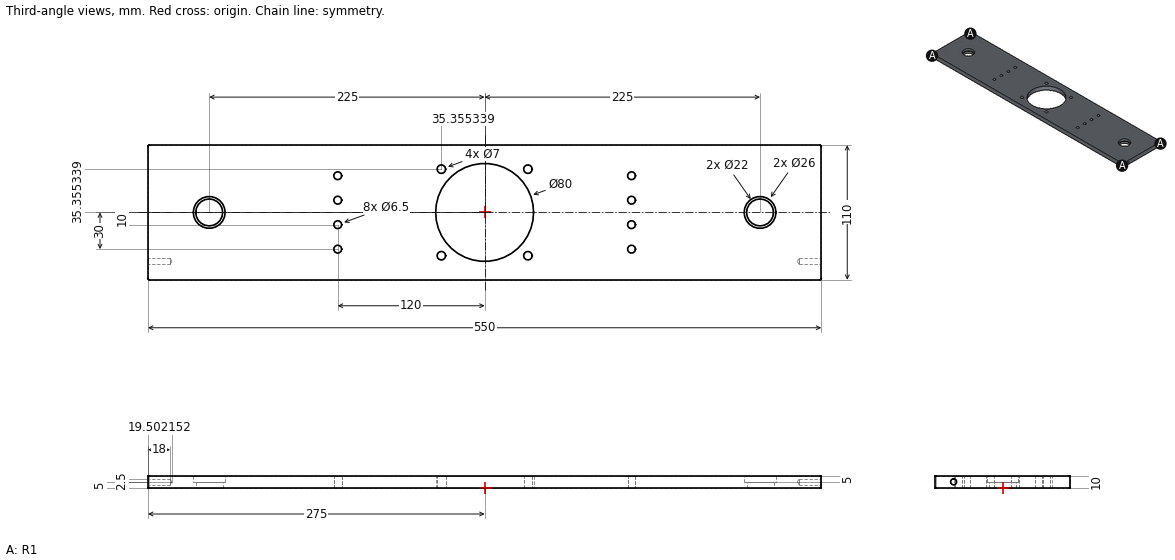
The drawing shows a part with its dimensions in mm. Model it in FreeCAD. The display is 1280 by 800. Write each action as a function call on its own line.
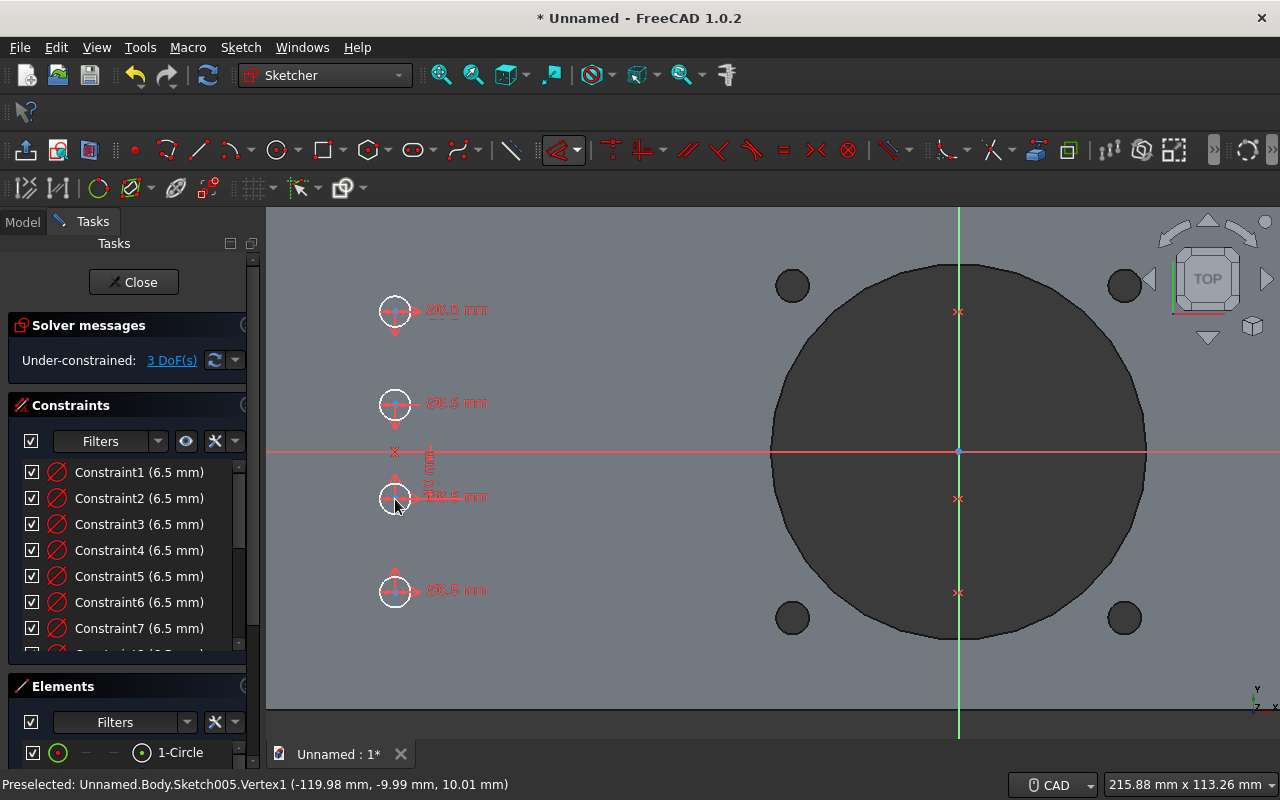
click(395, 592)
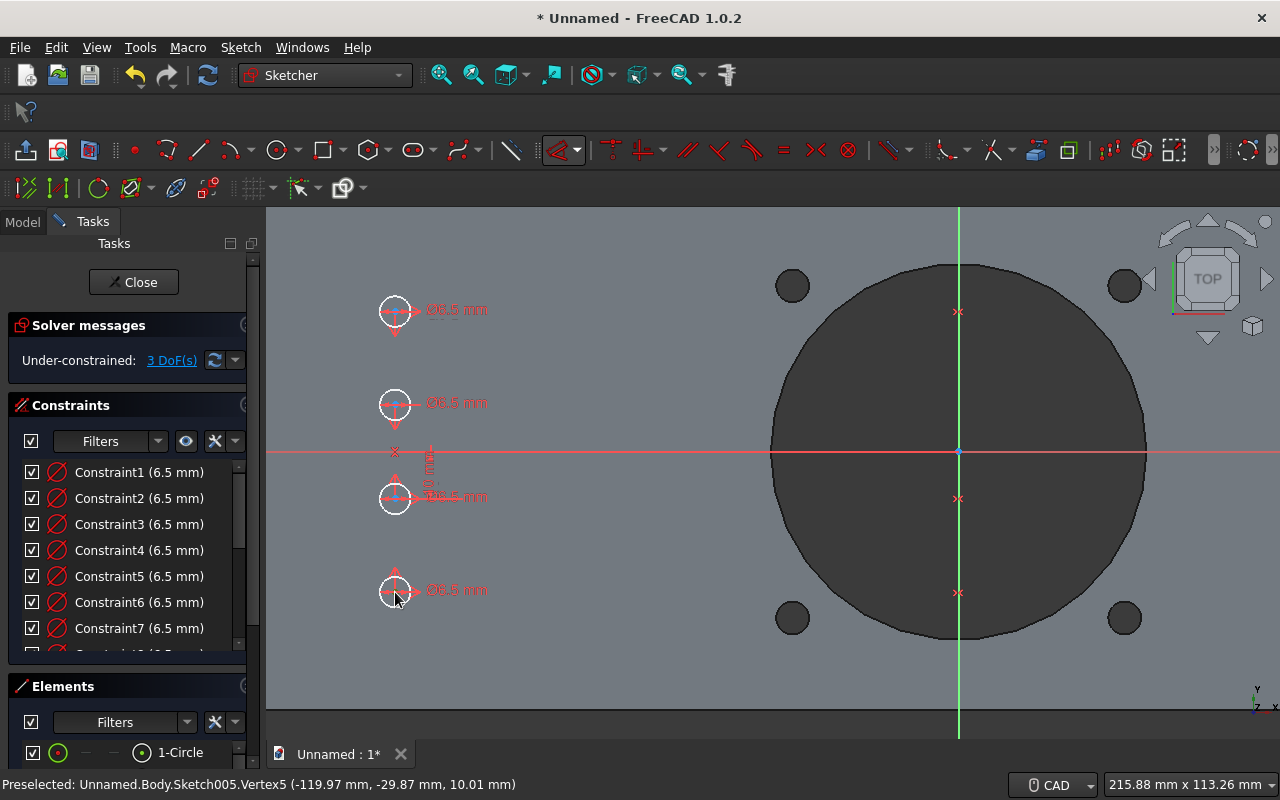
key(i)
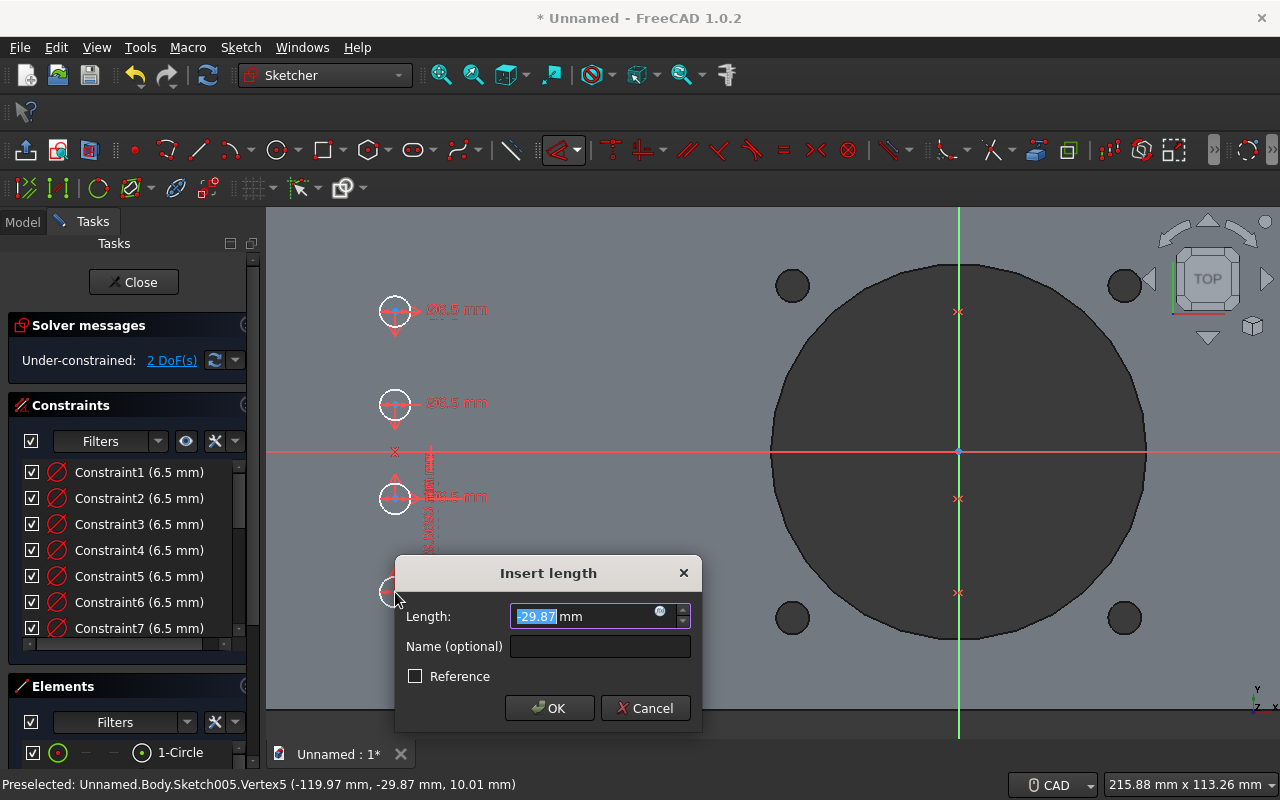
text(-30)
key(Return)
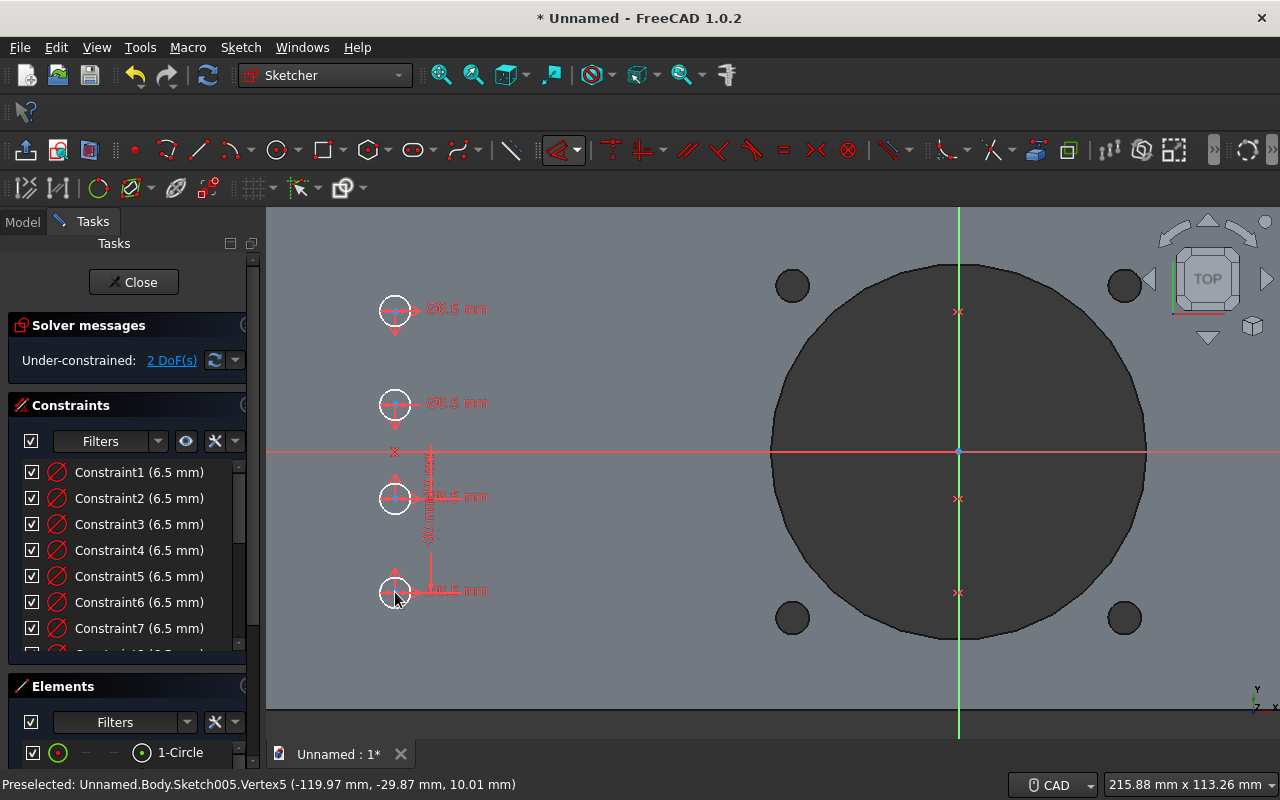
click(395, 499)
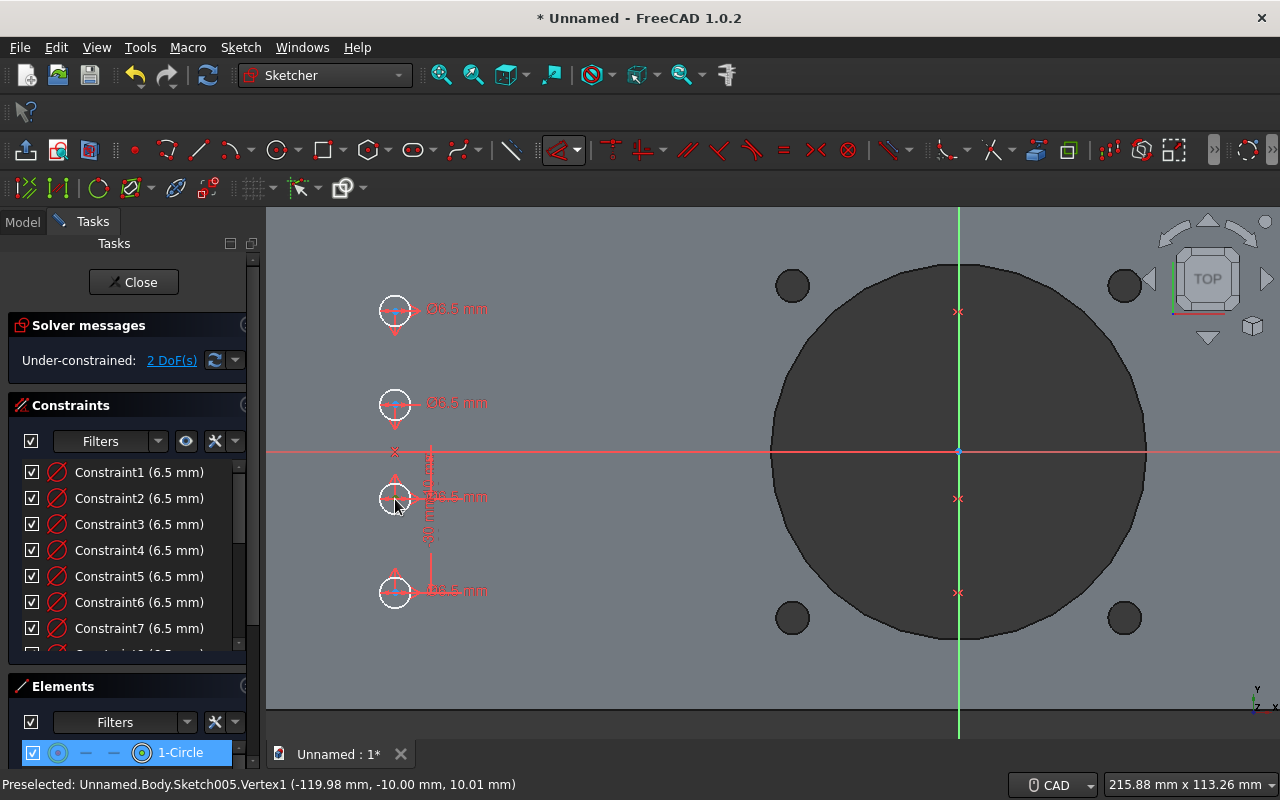
click(580, 150)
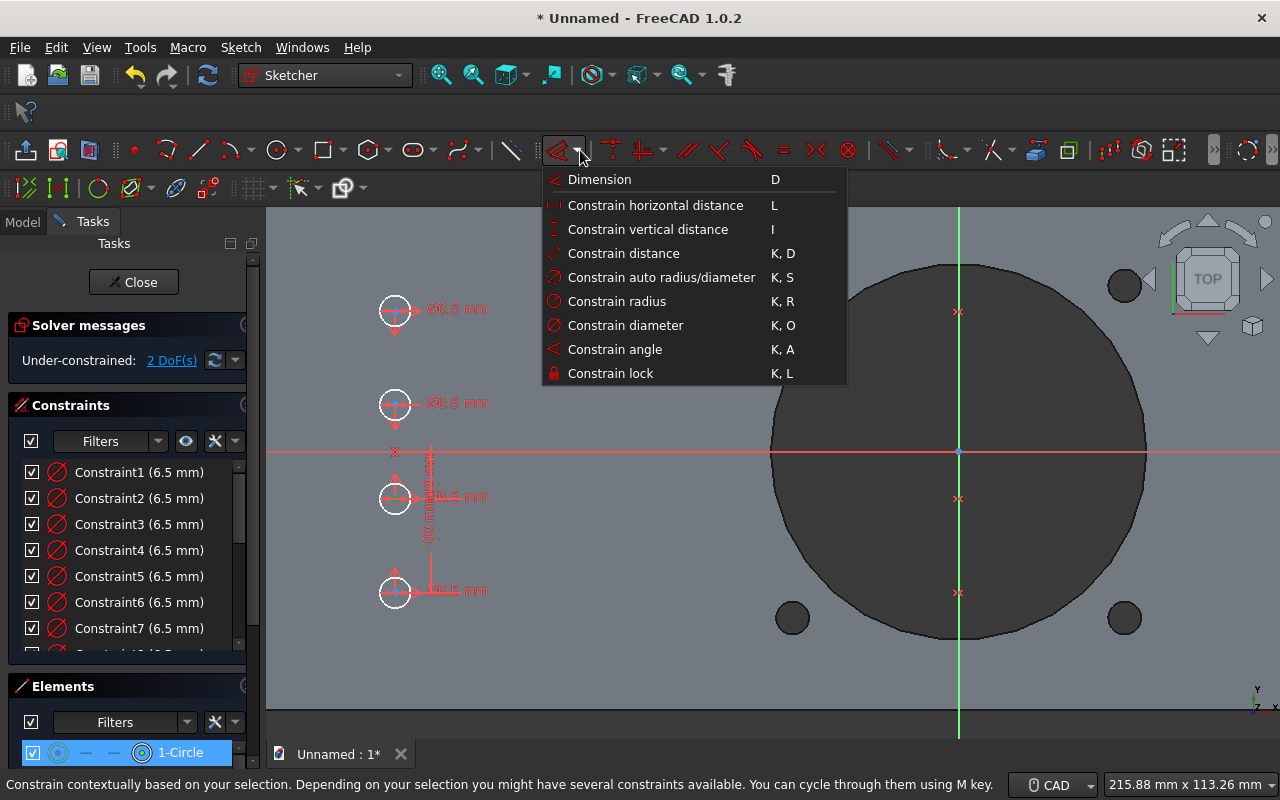
click(695, 205)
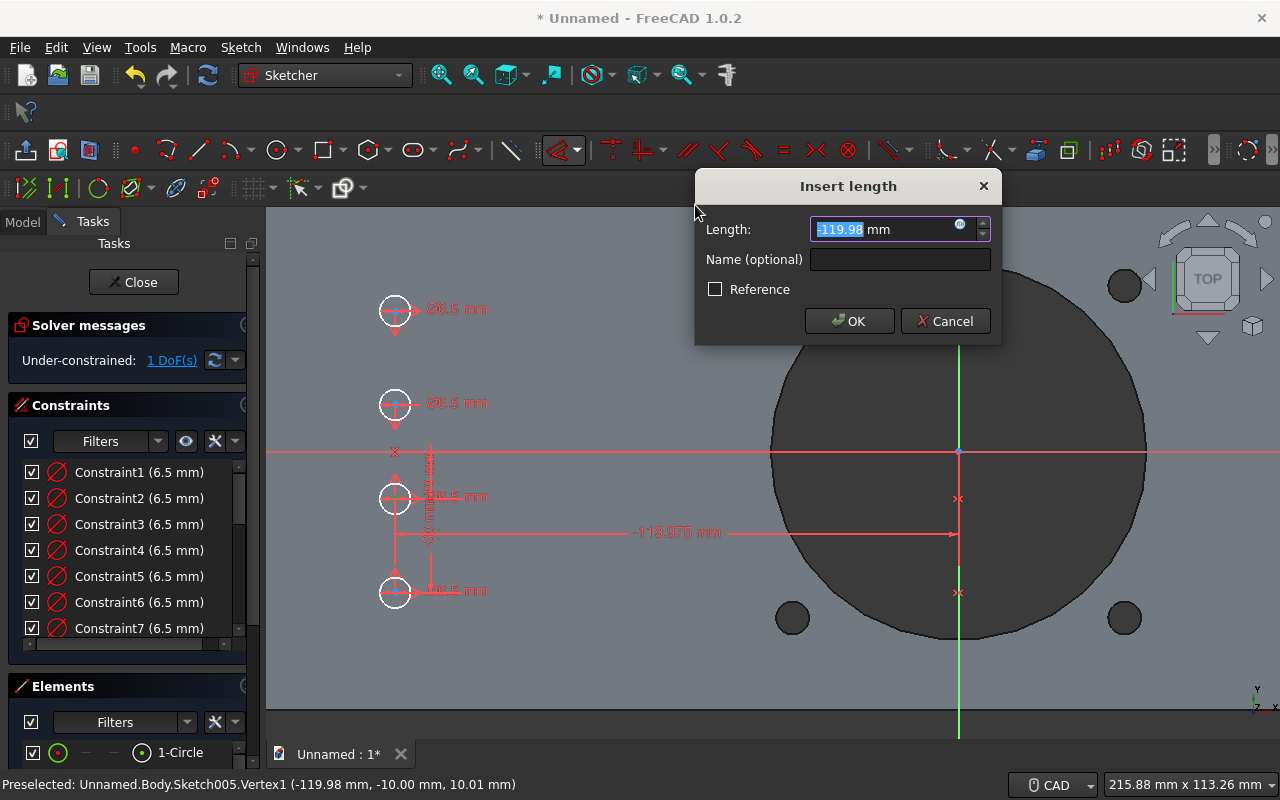
text(-120)
key(Return)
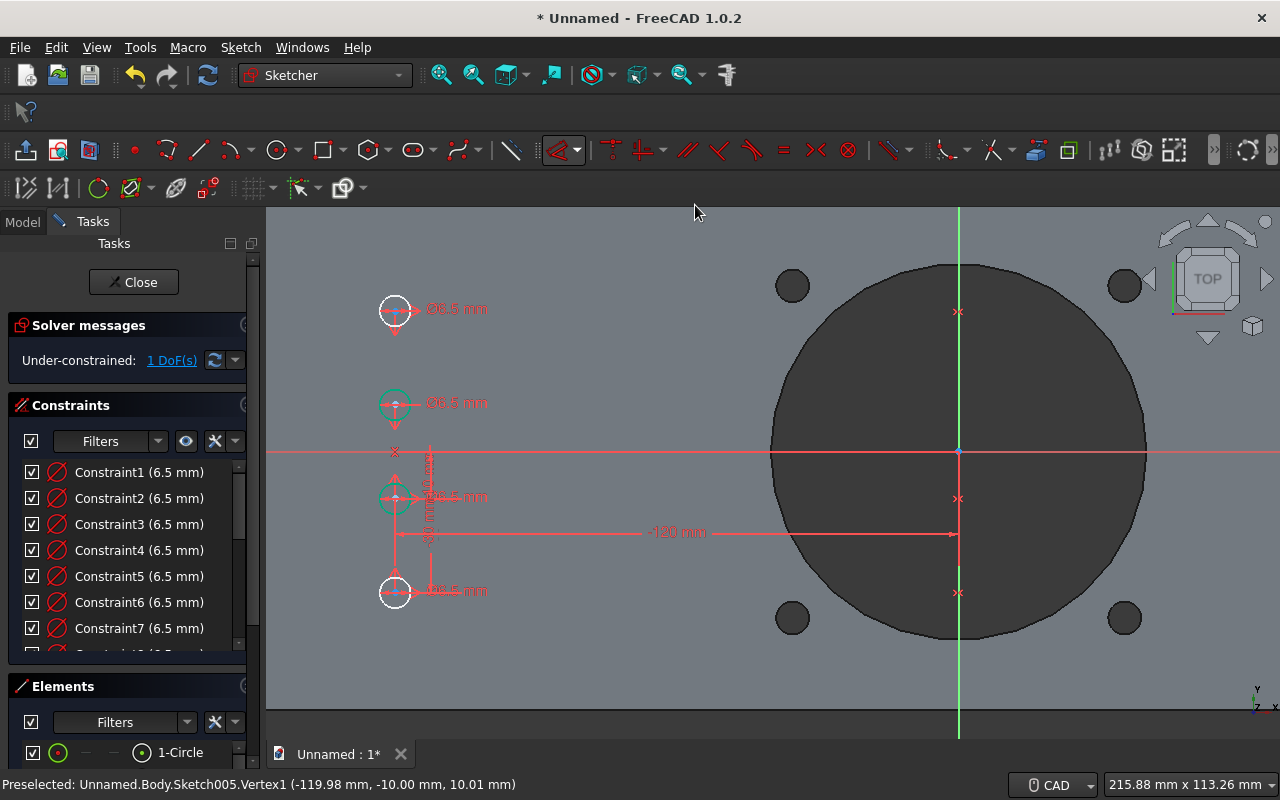
click(395, 593)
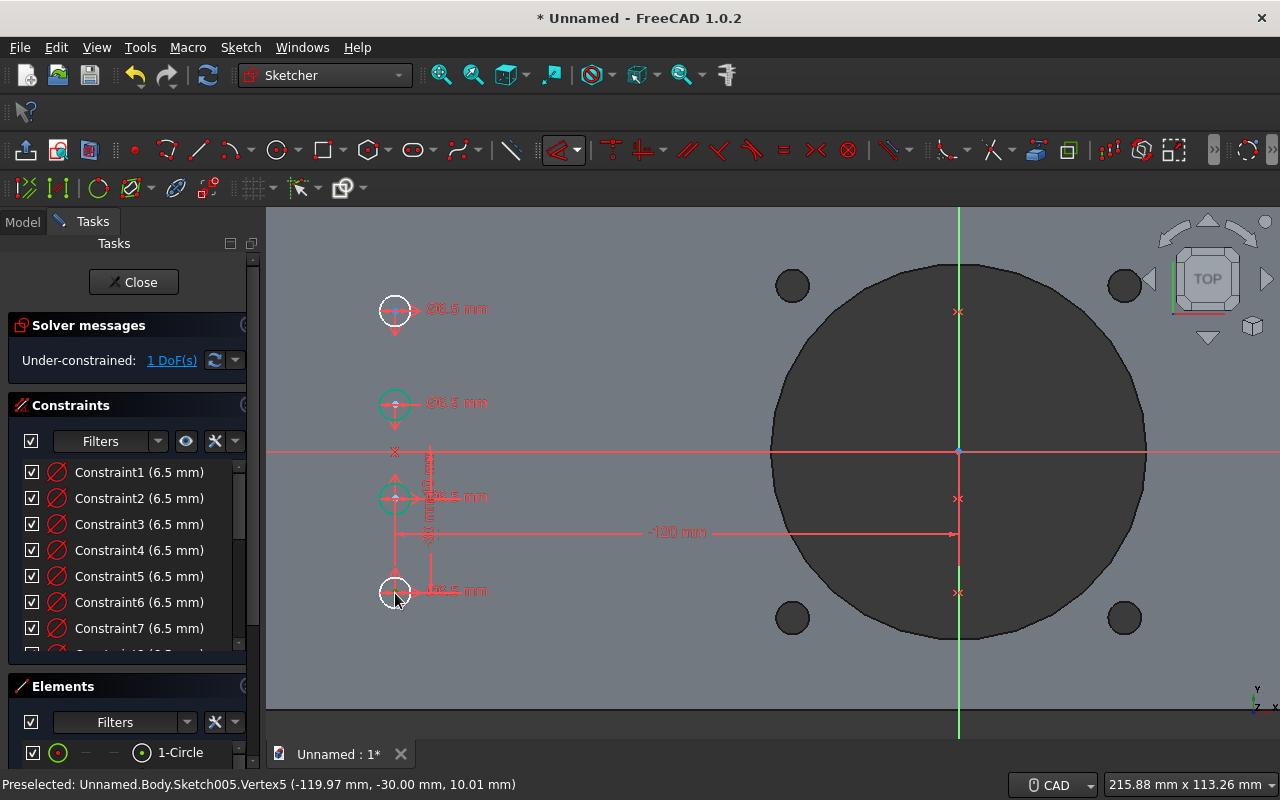
key(l)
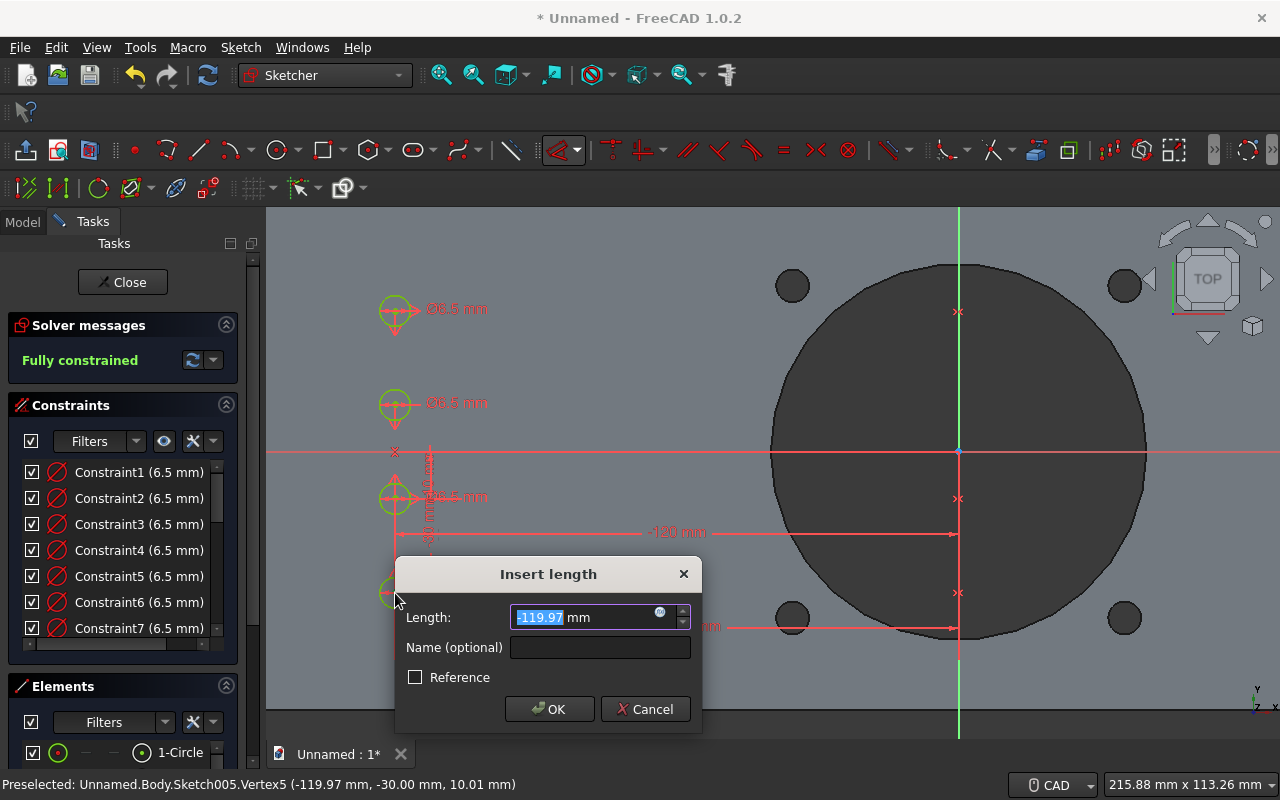
text(-120)
key(Return)